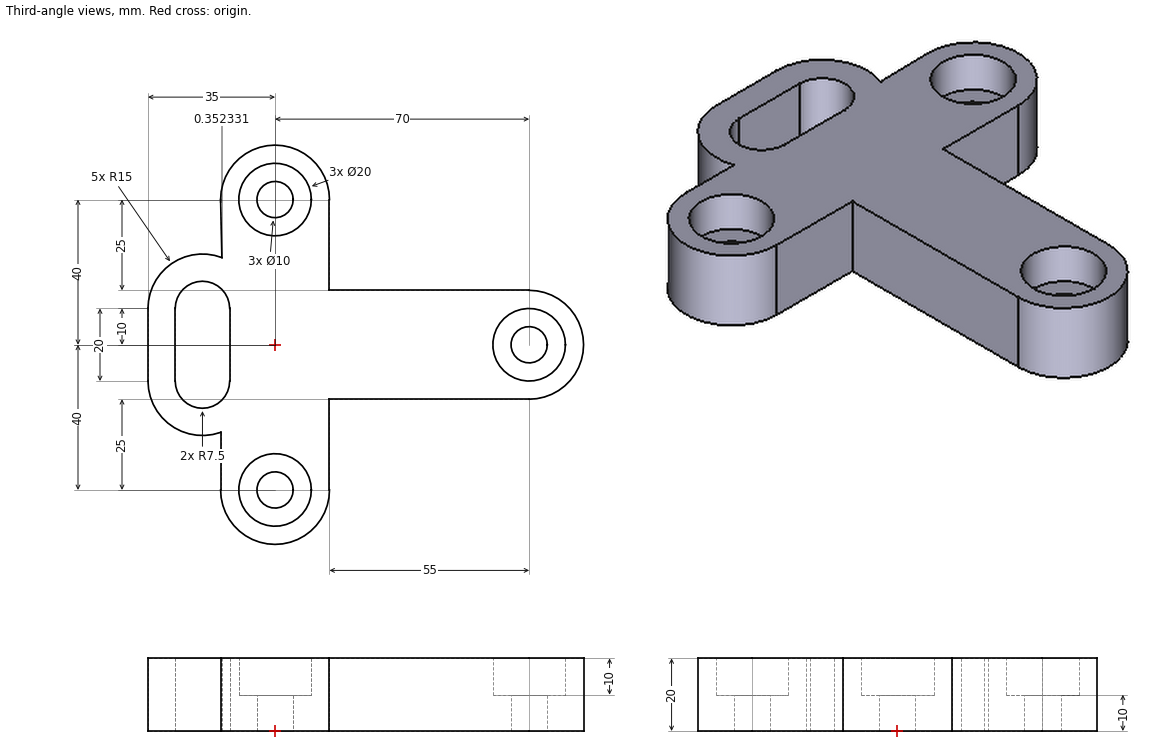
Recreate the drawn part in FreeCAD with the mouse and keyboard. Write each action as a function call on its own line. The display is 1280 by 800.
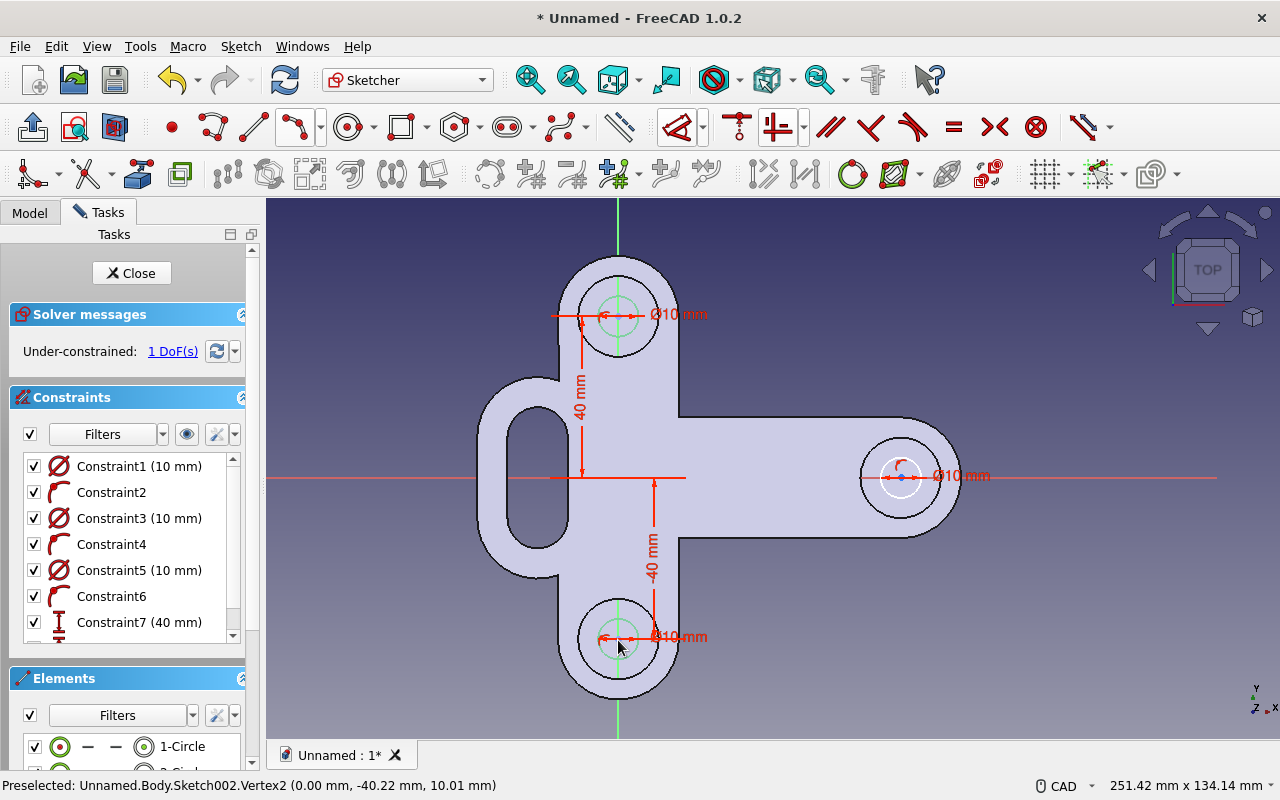
click(901, 478)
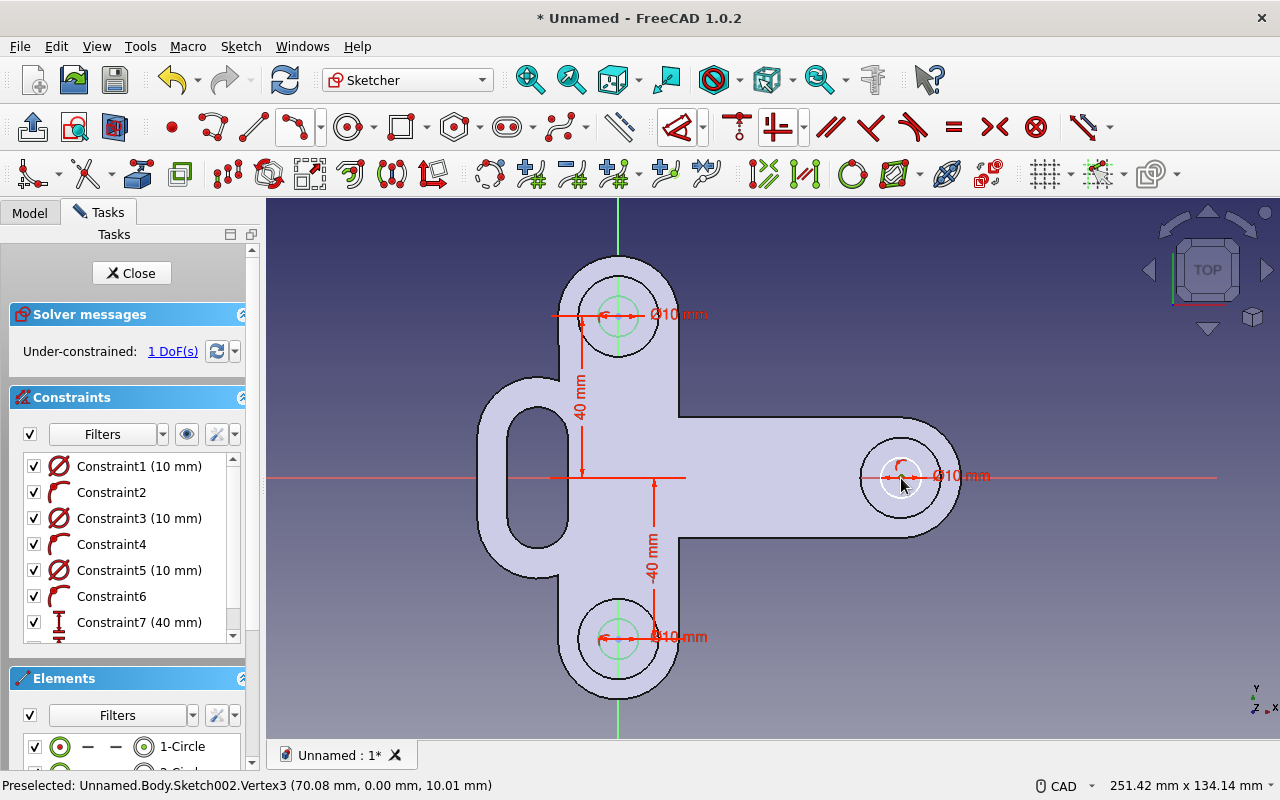
click(702, 128)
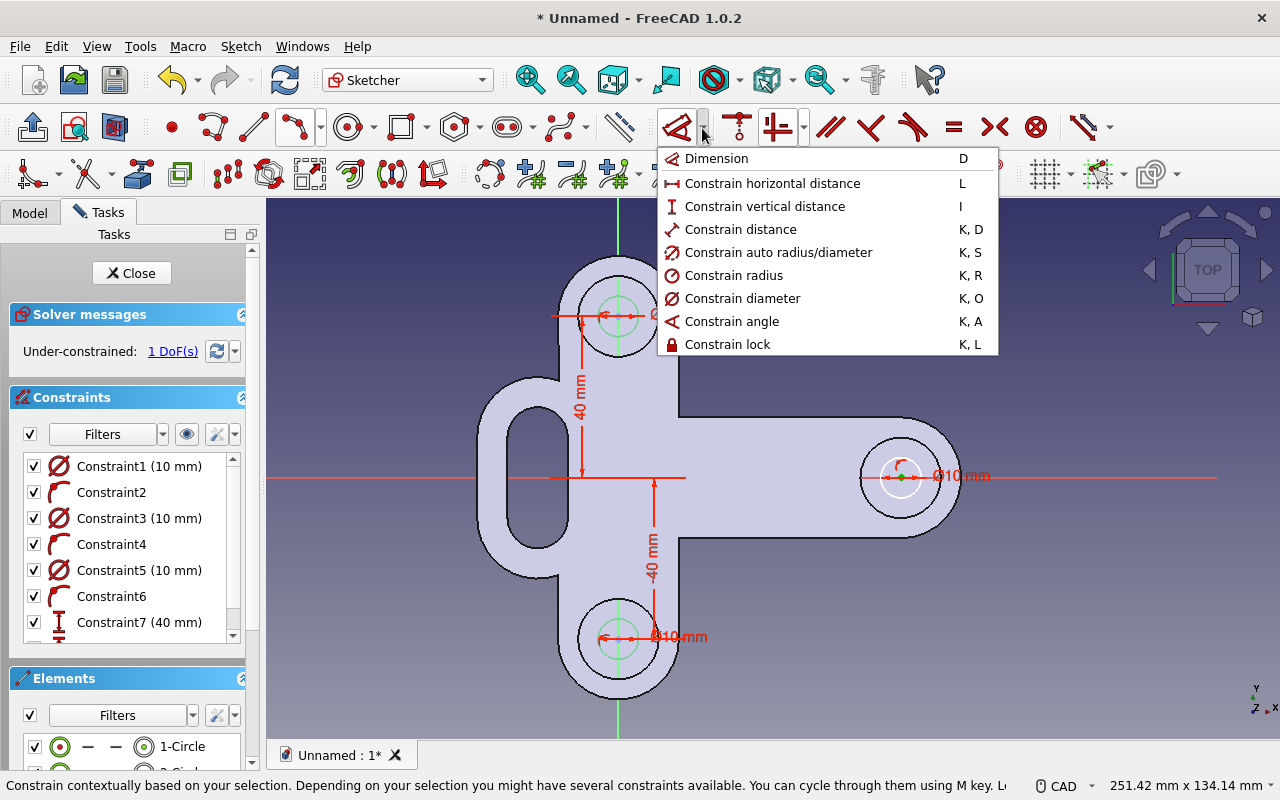
click(828, 184)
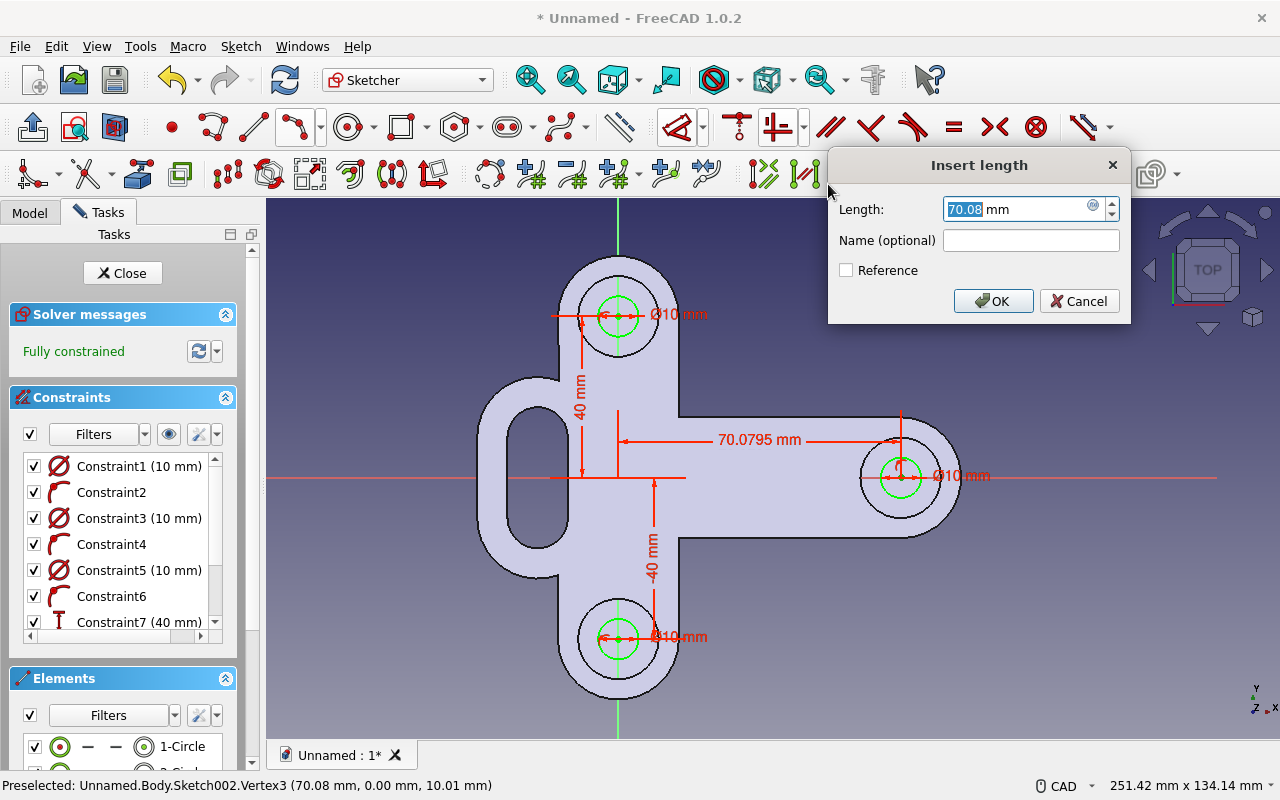
text(70)
key(Return)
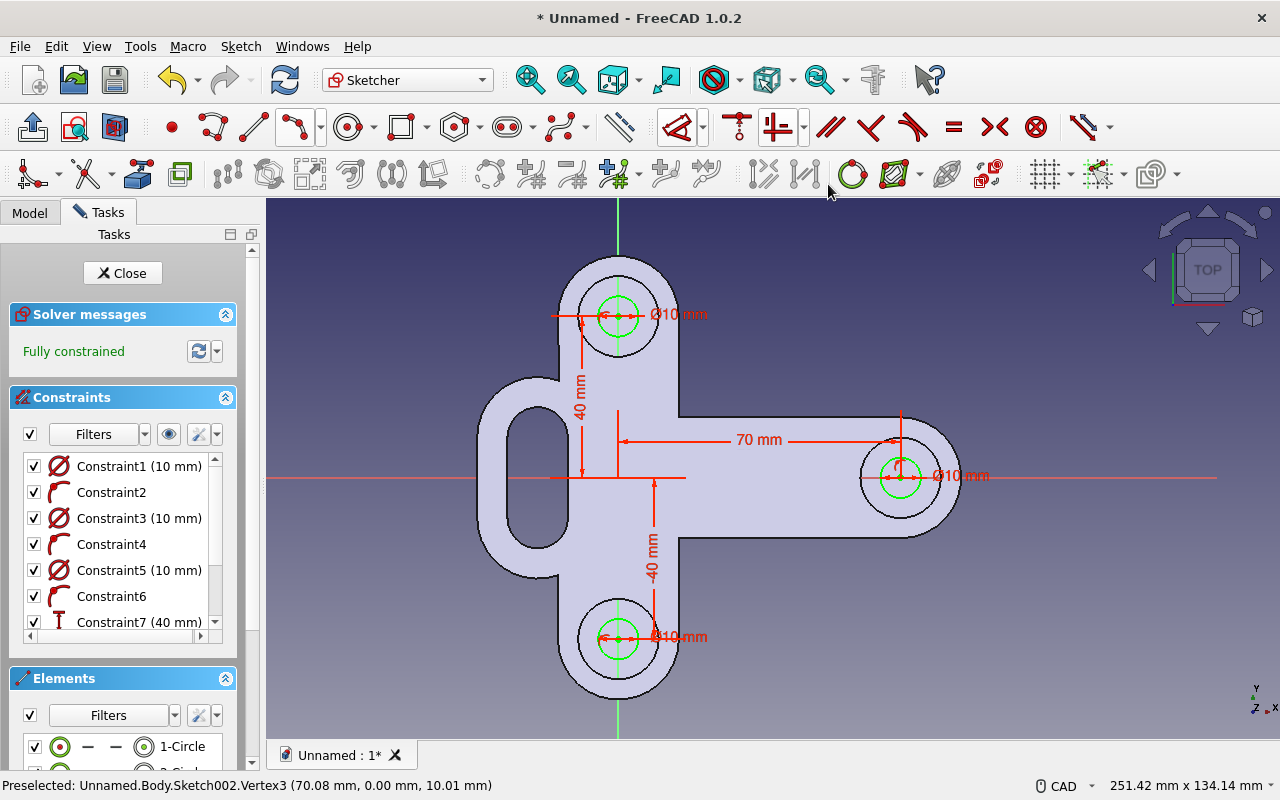
click(123, 273)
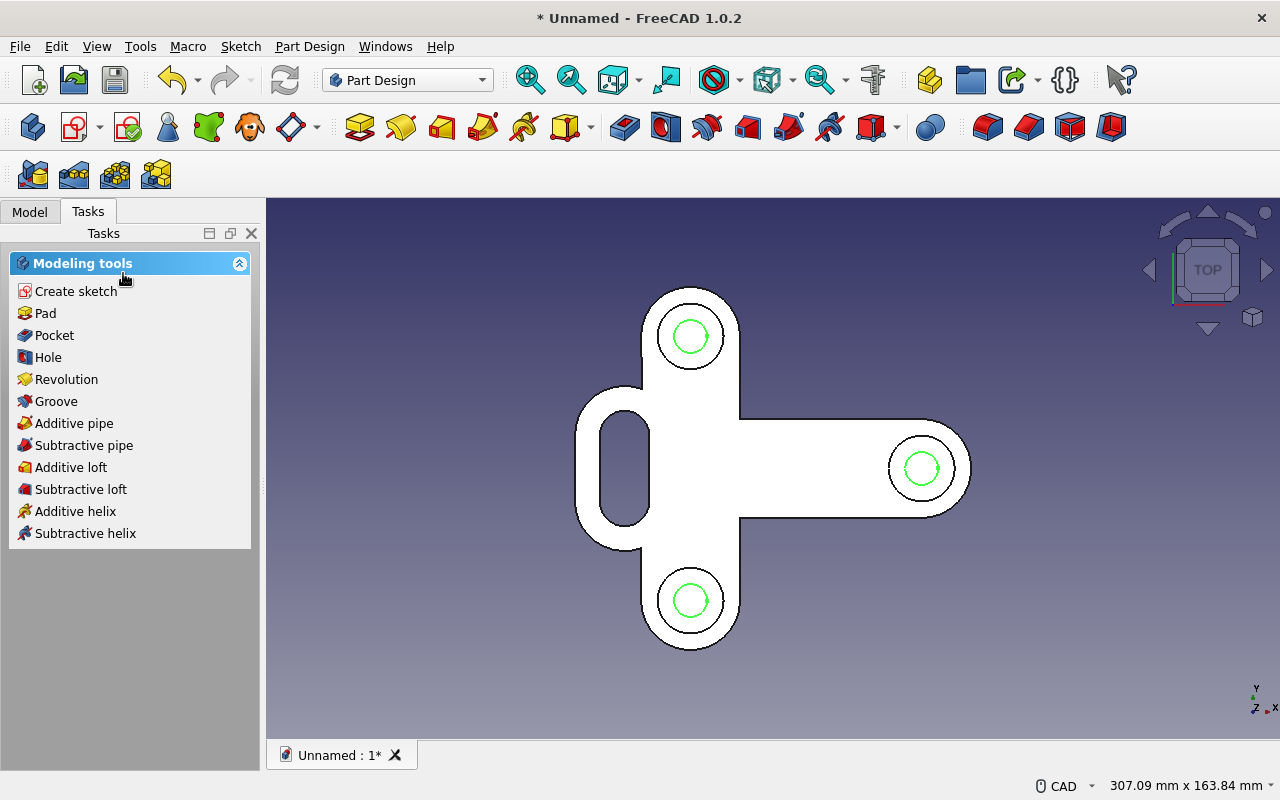
click(625, 128)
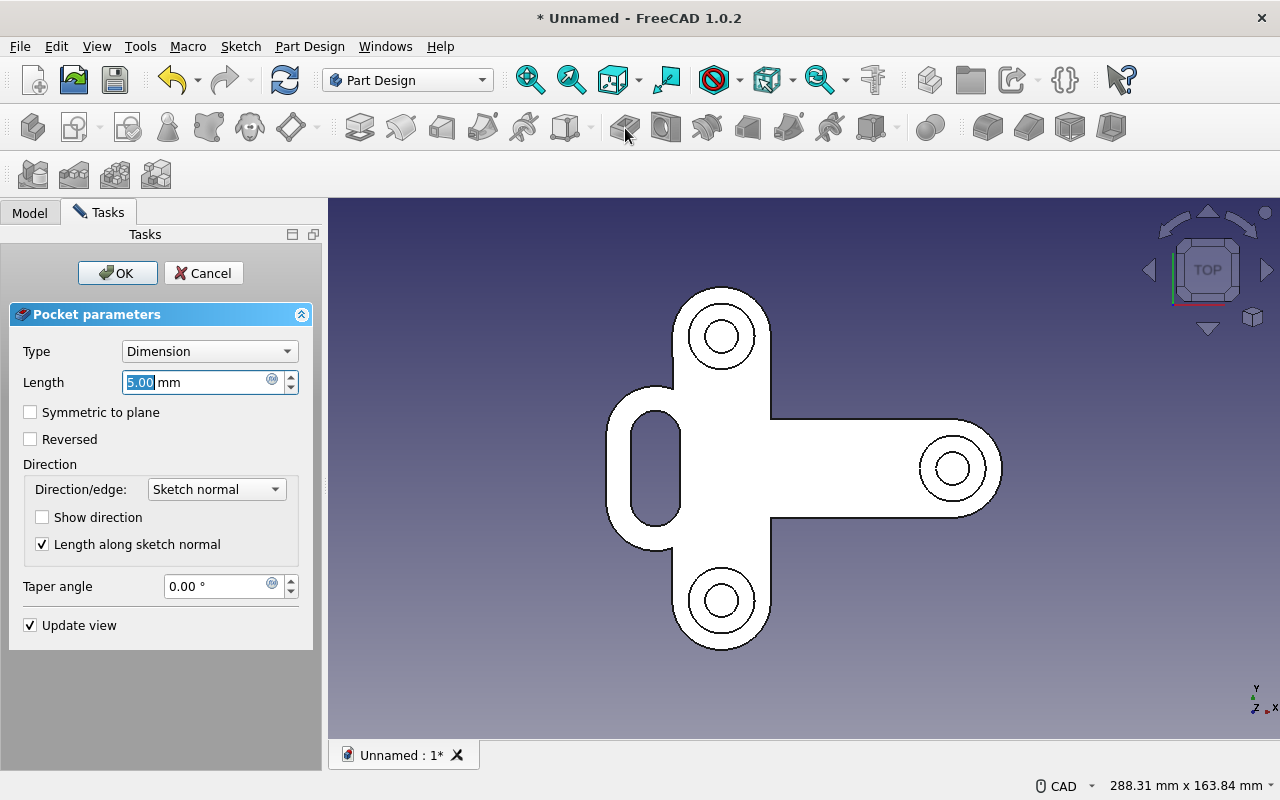
text(10)
key(Tab)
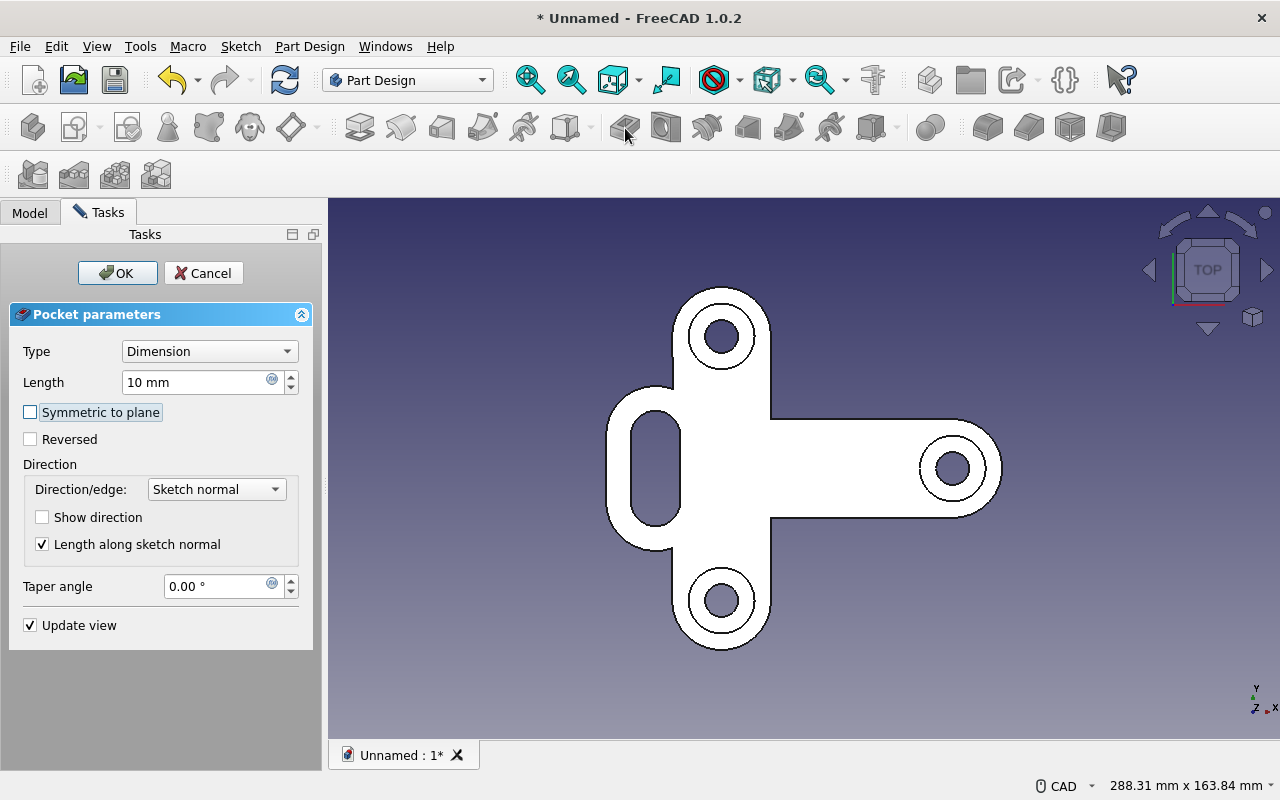
click(118, 273)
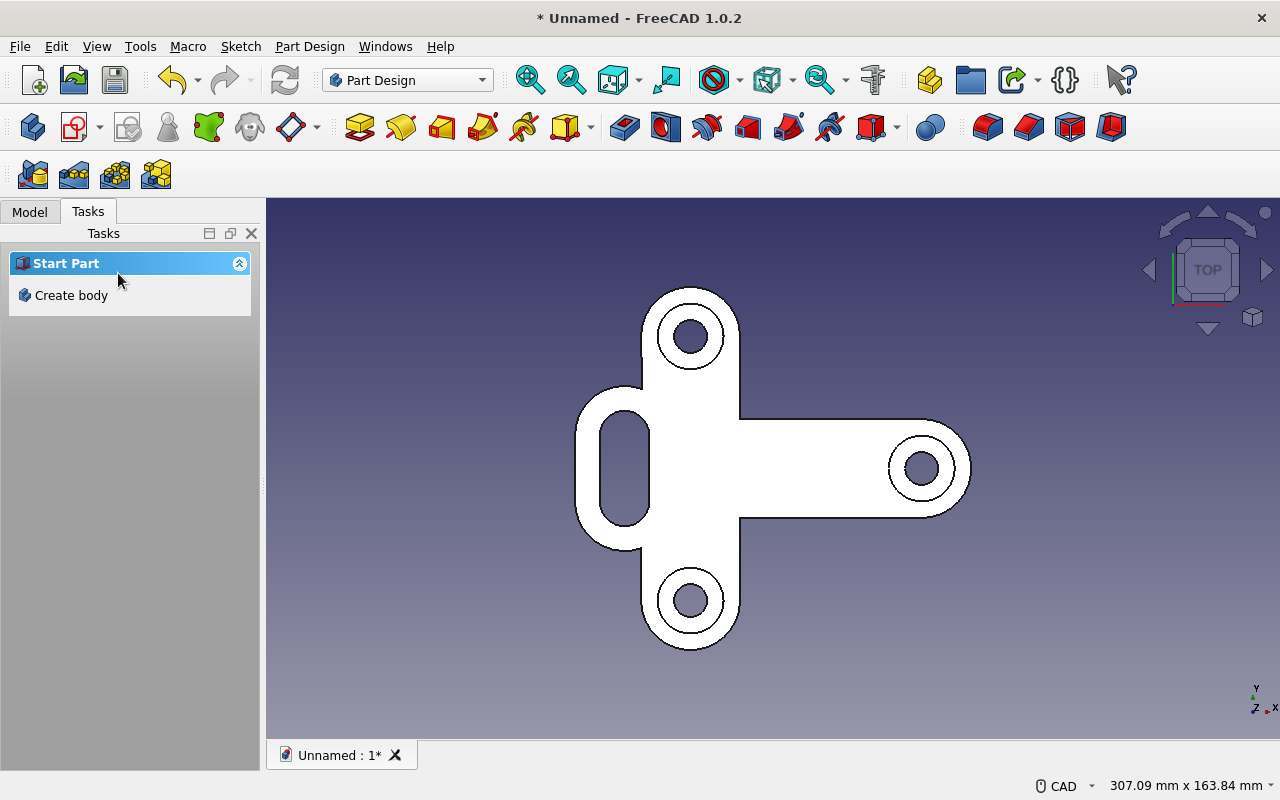
key(0)